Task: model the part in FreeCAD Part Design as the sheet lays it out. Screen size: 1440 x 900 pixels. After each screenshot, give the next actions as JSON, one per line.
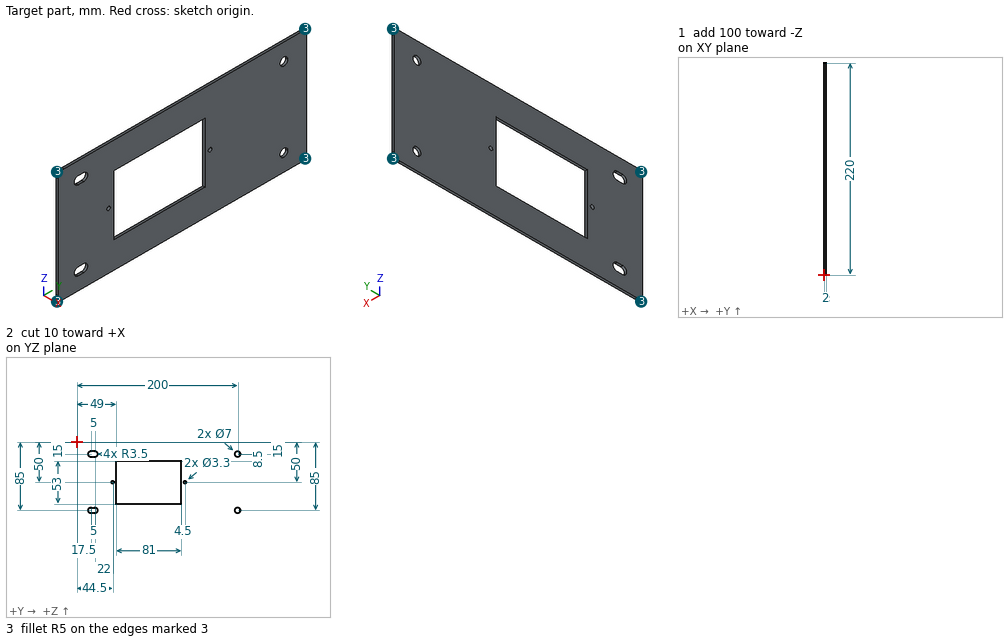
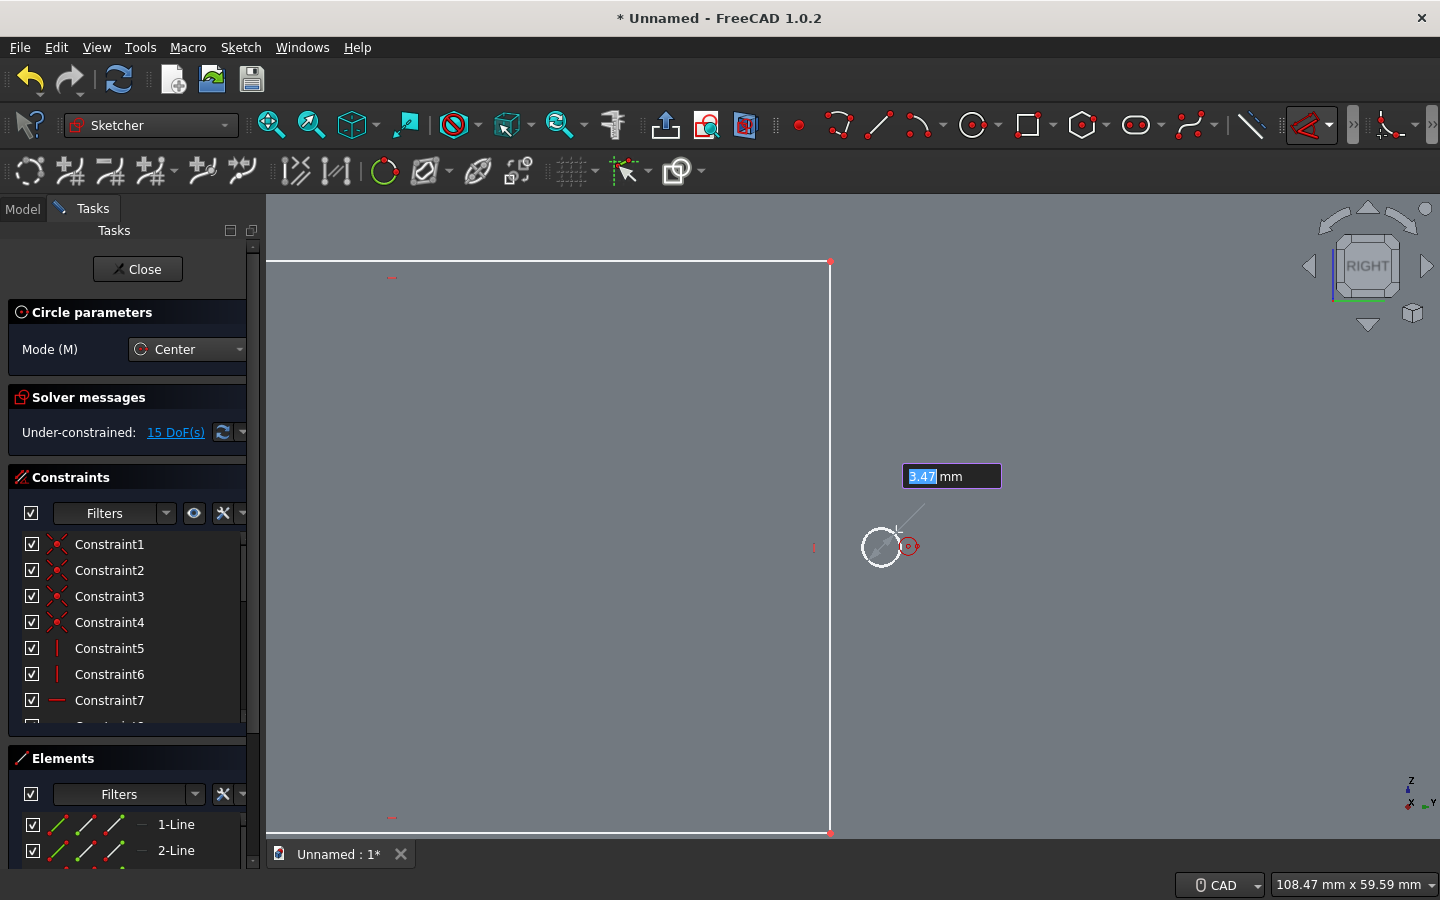
{"action": "left_click", "coordinate": [893, 531]}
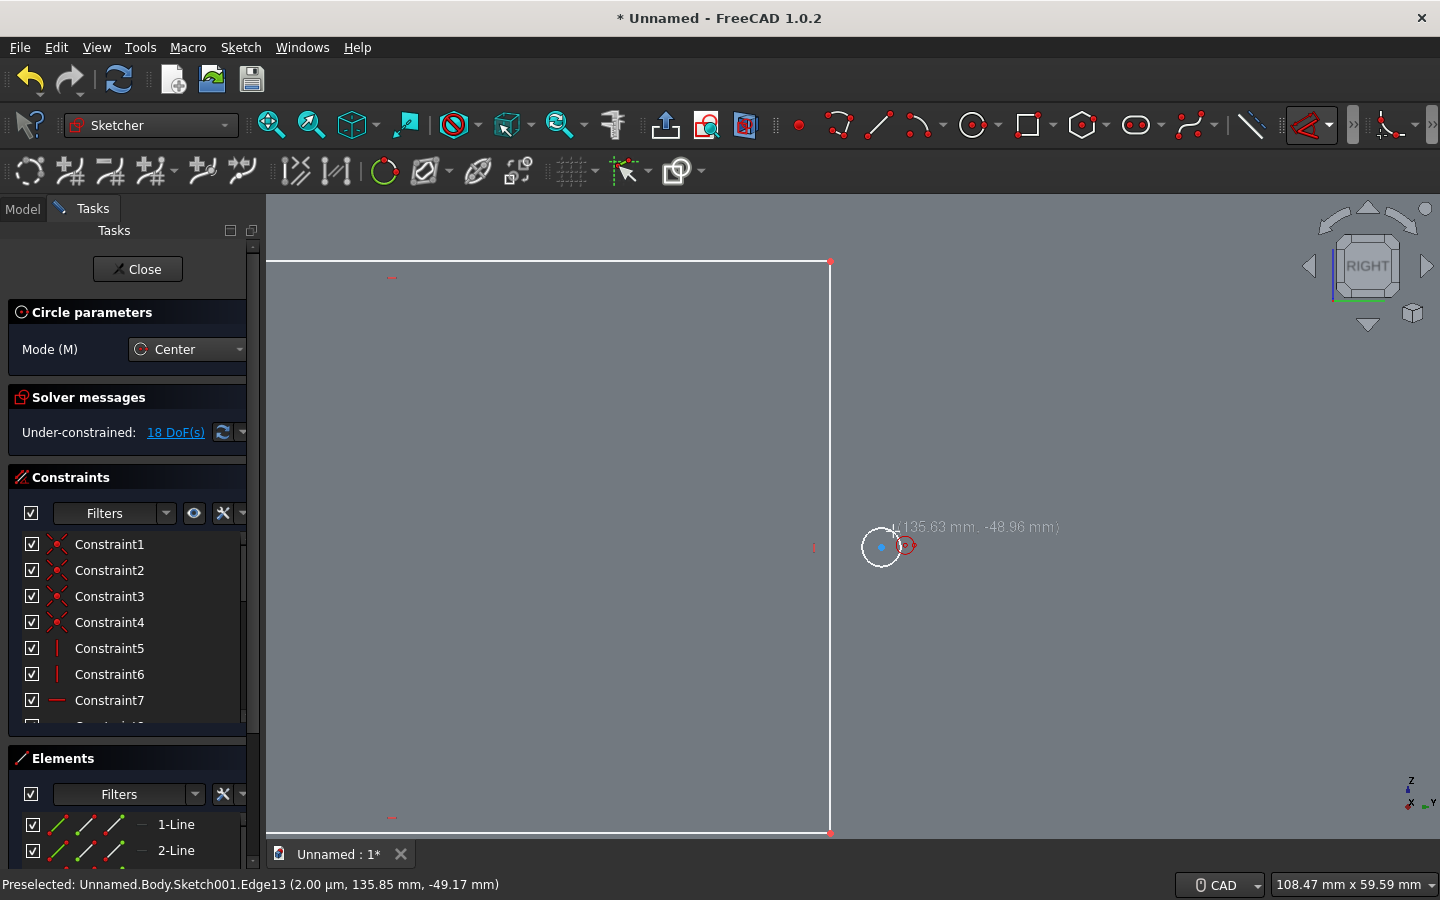
{"action": "scroll", "coordinate": [896, 532], "scroll_direction": "down", "scroll_amount": 6}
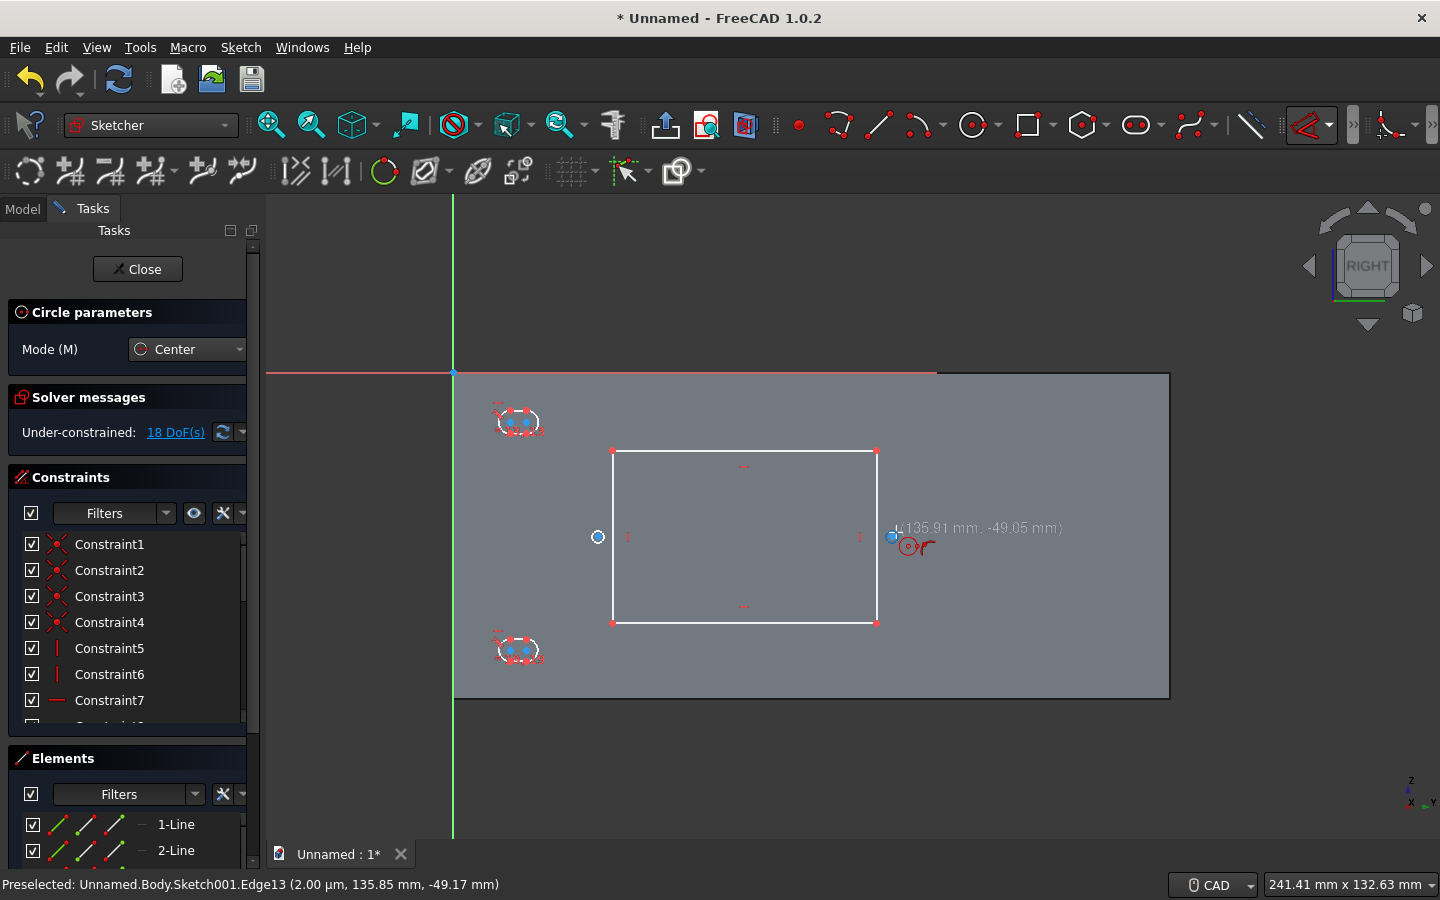
{"action": "scroll", "coordinate": [1105, 422], "scroll_direction": "up", "scroll_amount": 4}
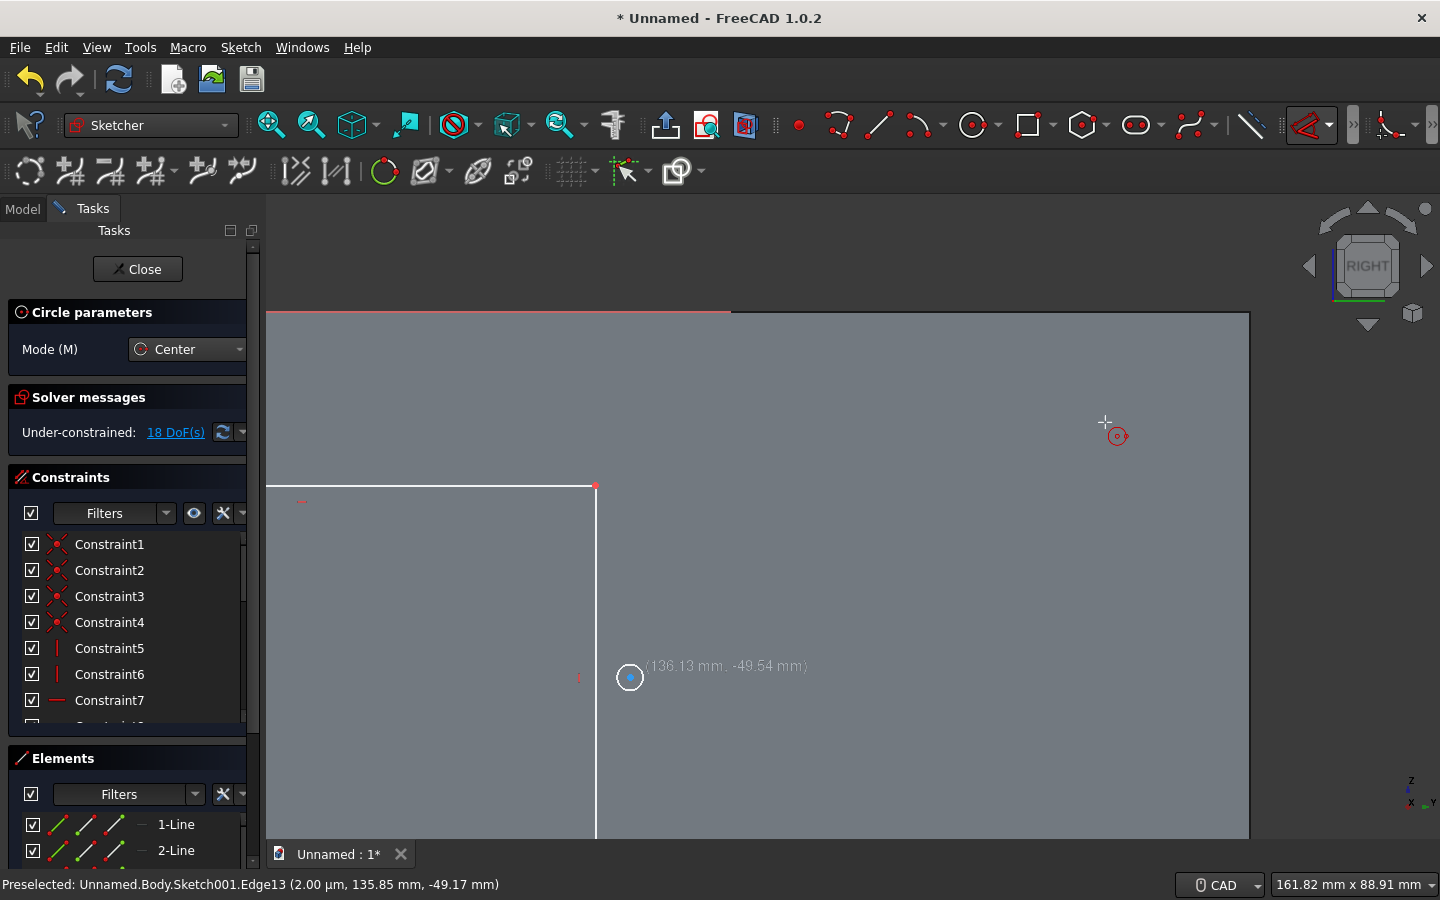
{"action": "left_click", "coordinate": [1105, 421]}
{"action": "left_click", "coordinate": [1123, 403]}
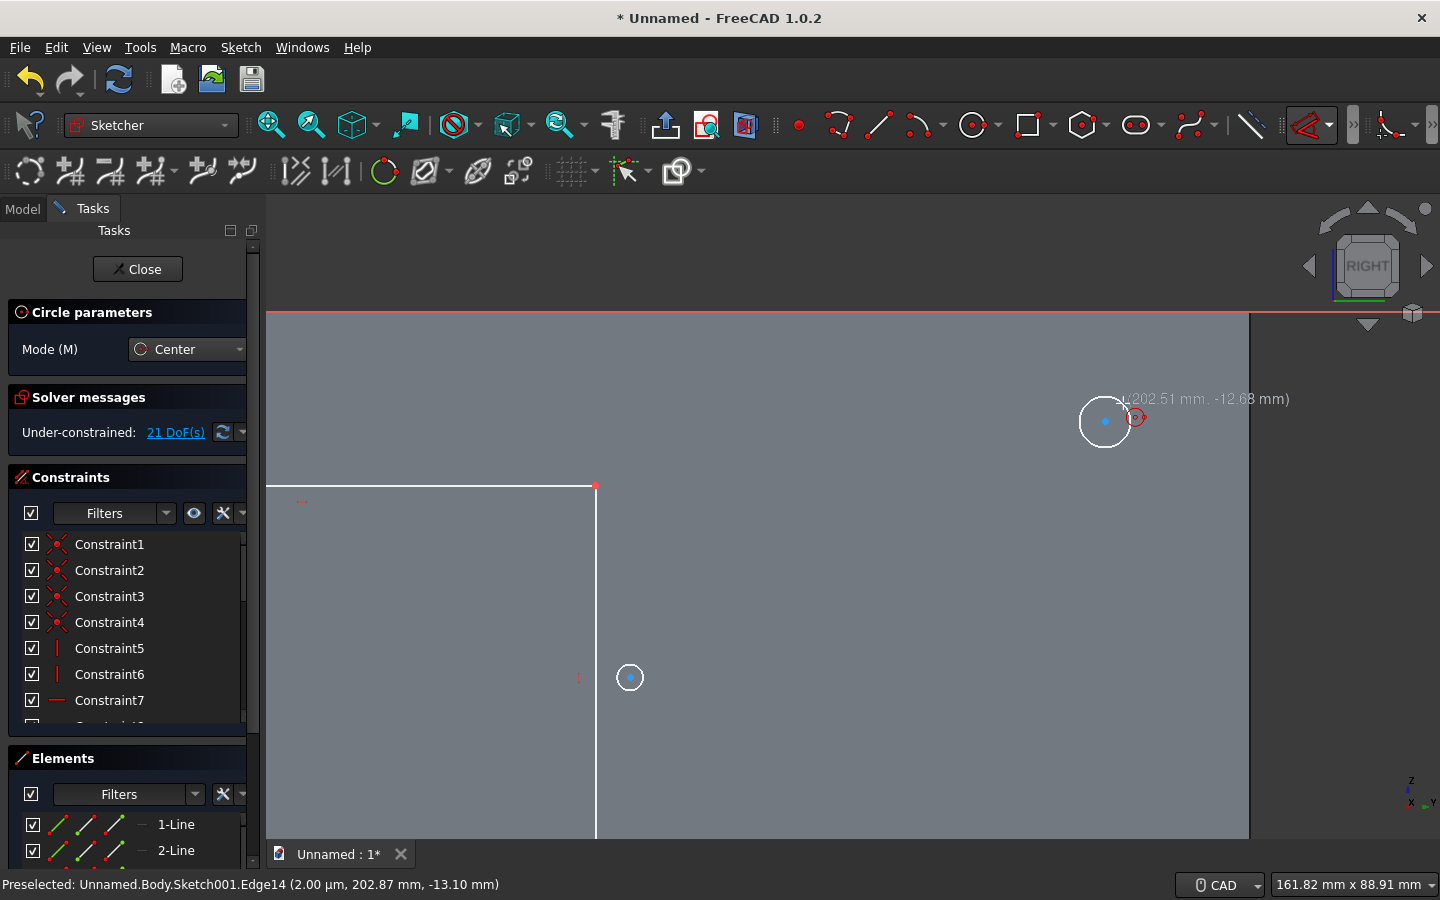
{"action": "scroll", "coordinate": [1105, 421], "scroll_direction": "down", "scroll_amount": 4}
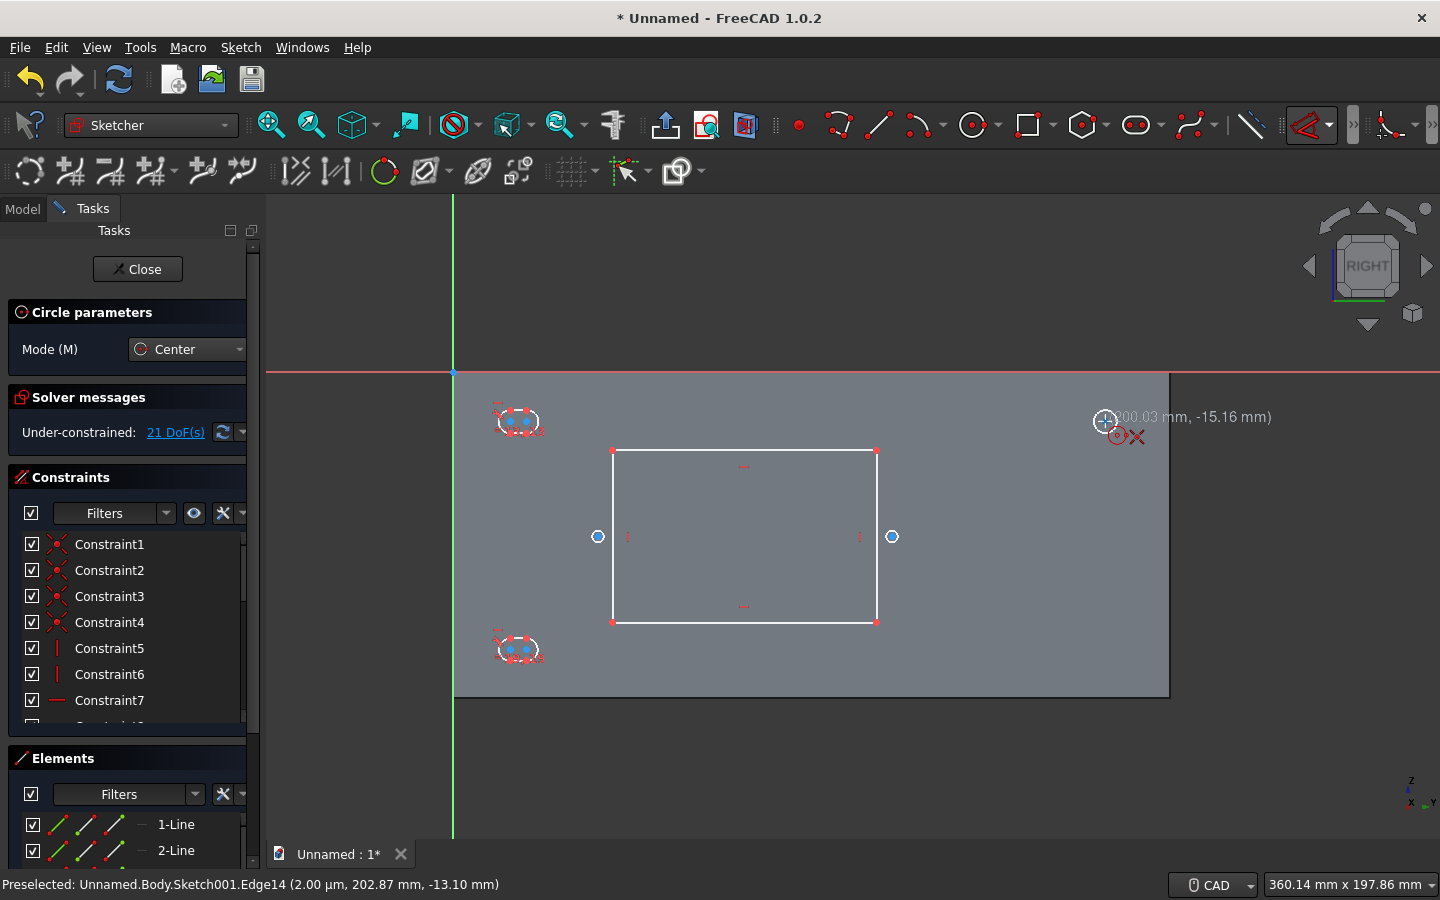
{"action": "scroll", "coordinate": [1105, 649], "scroll_direction": "up", "scroll_amount": 4}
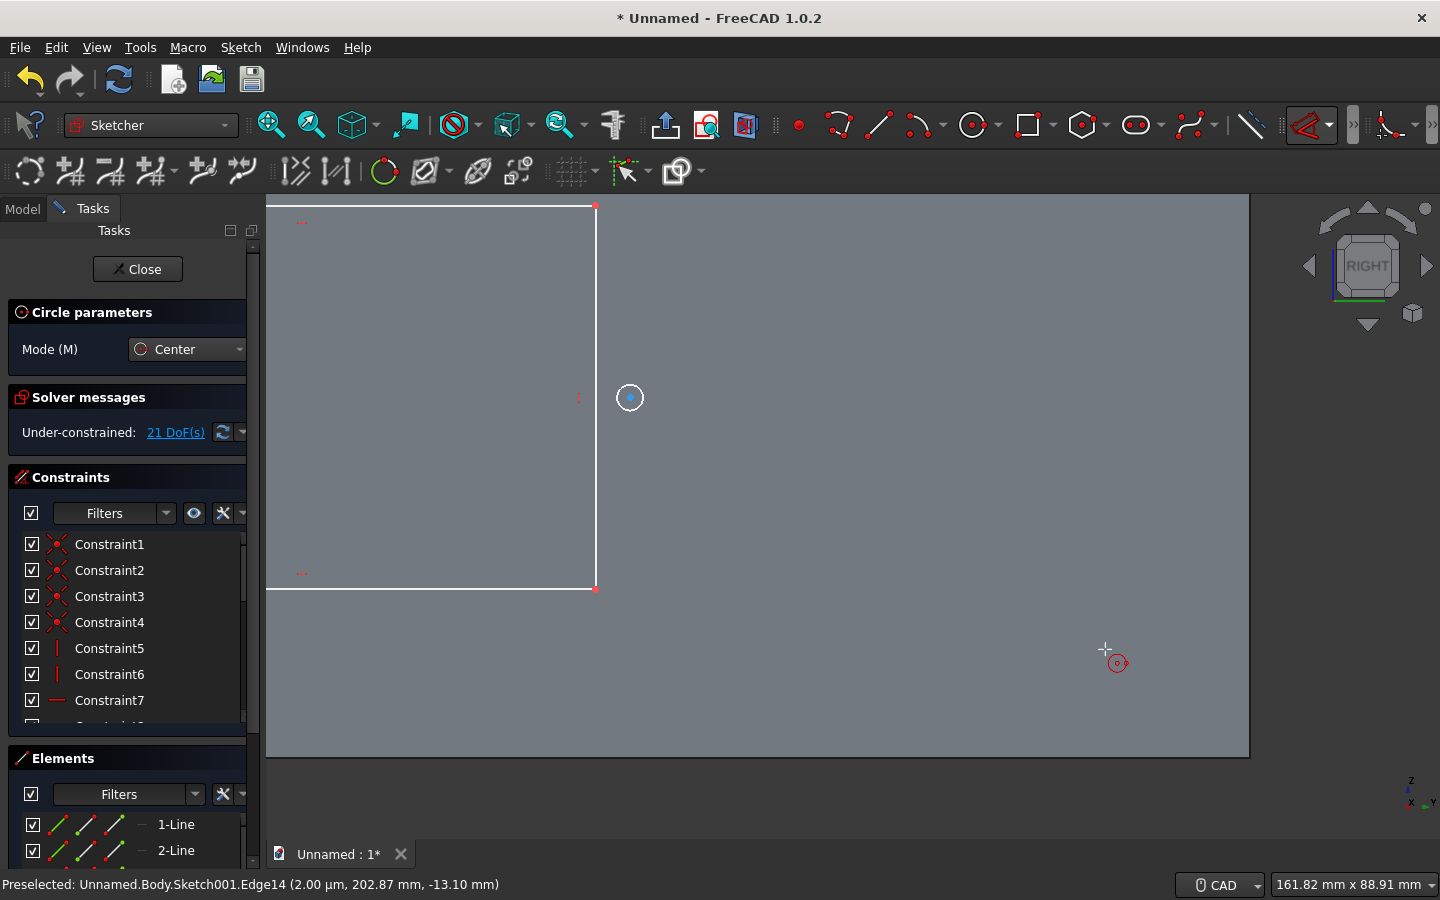
{"action": "left_click", "coordinate": [1105, 649]}
{"action": "left_click", "coordinate": [1123, 631]}
{"action": "key", "text": "Escape"}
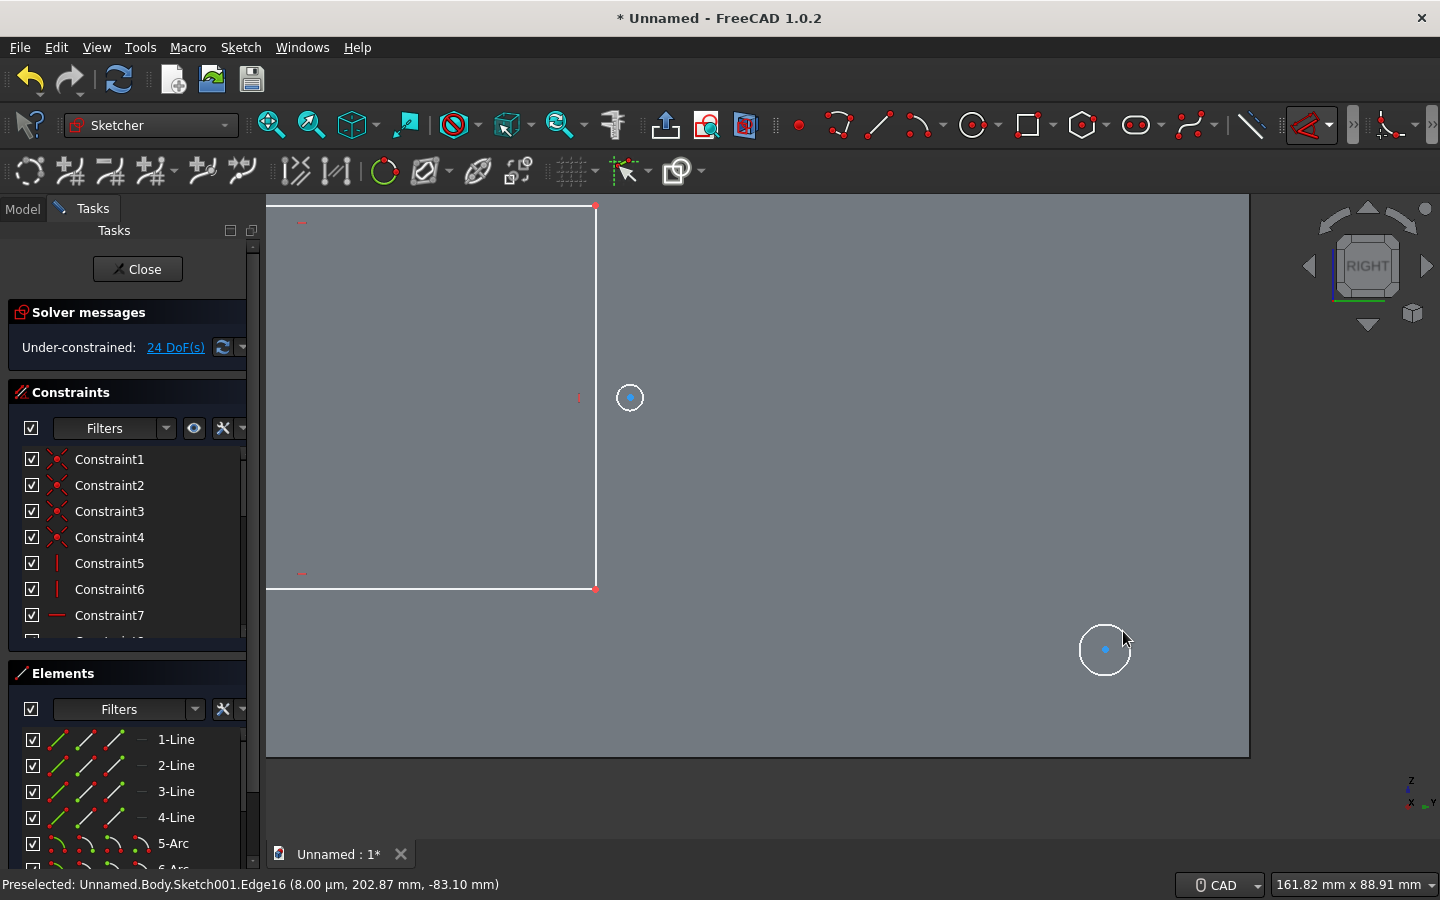
{"action": "scroll", "coordinate": [1105, 650], "scroll_direction": "down", "scroll_amount": 4}